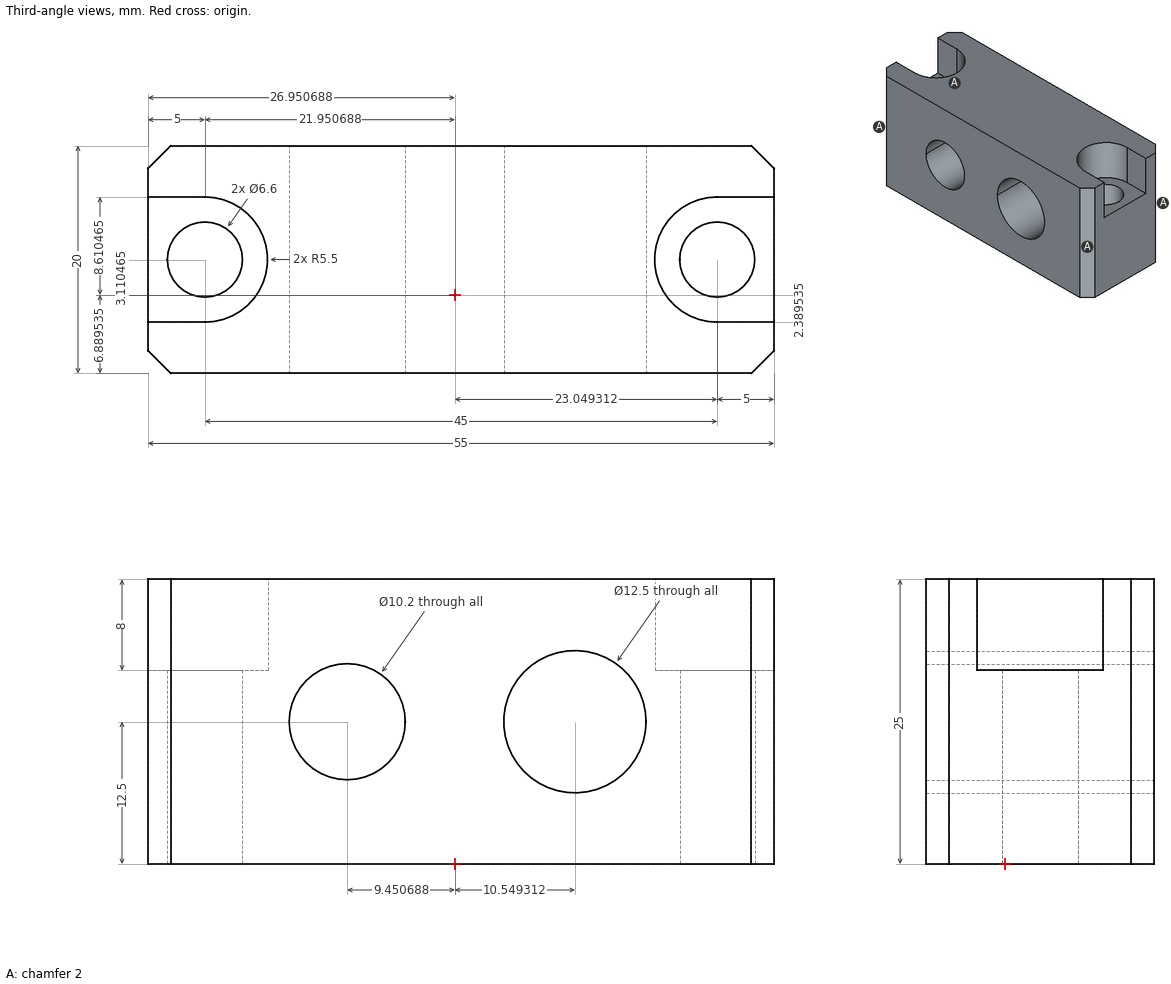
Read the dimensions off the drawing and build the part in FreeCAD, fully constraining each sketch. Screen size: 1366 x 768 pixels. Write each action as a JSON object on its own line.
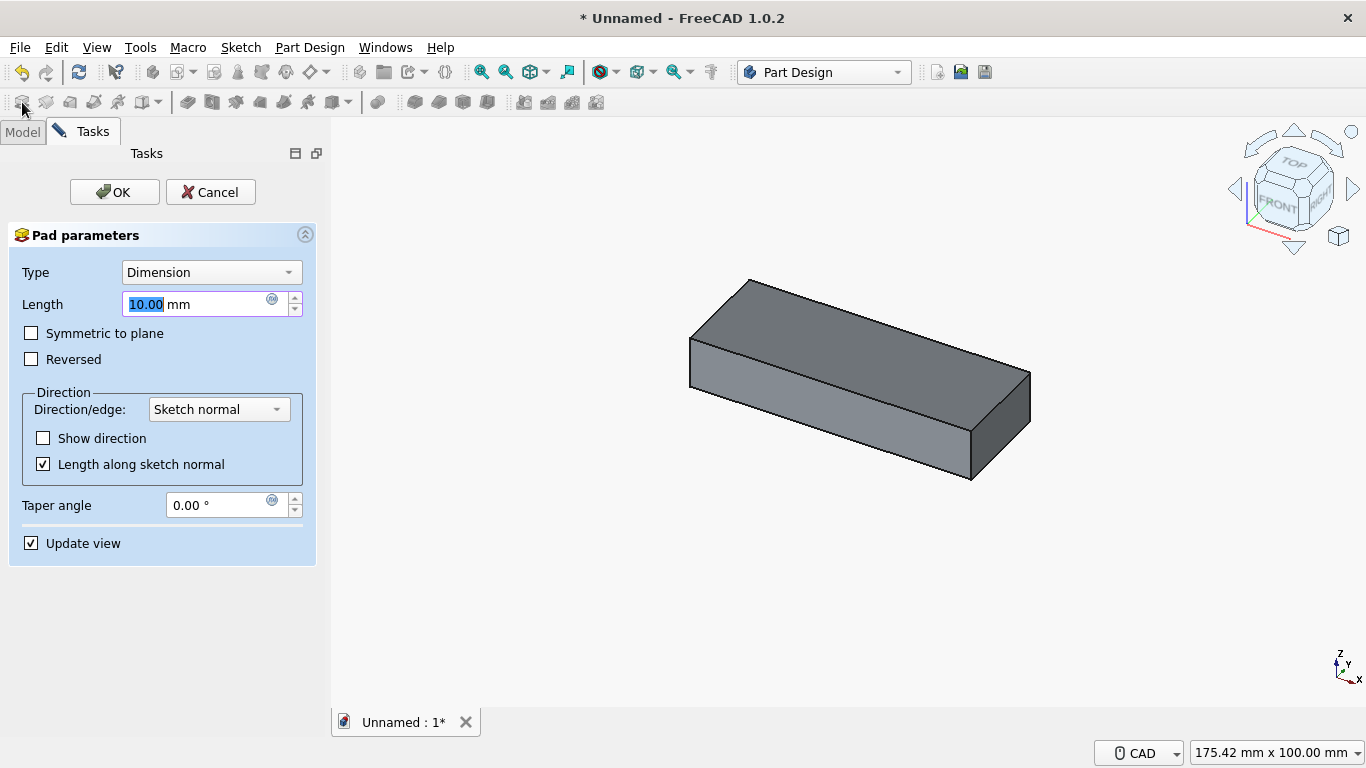
{"action": "type", "text": "25"}
{"action": "key", "text": "Tab"}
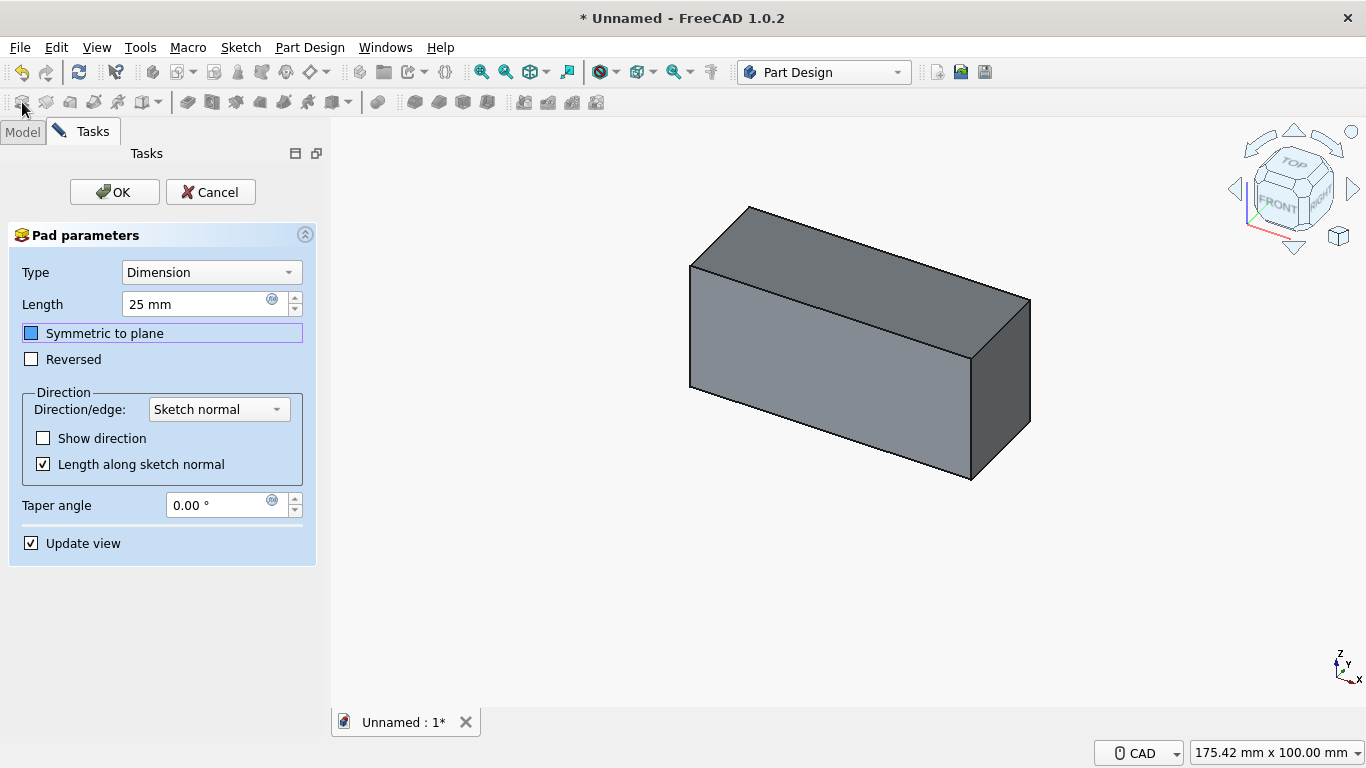
{"action": "left_click", "coordinate": [115, 192]}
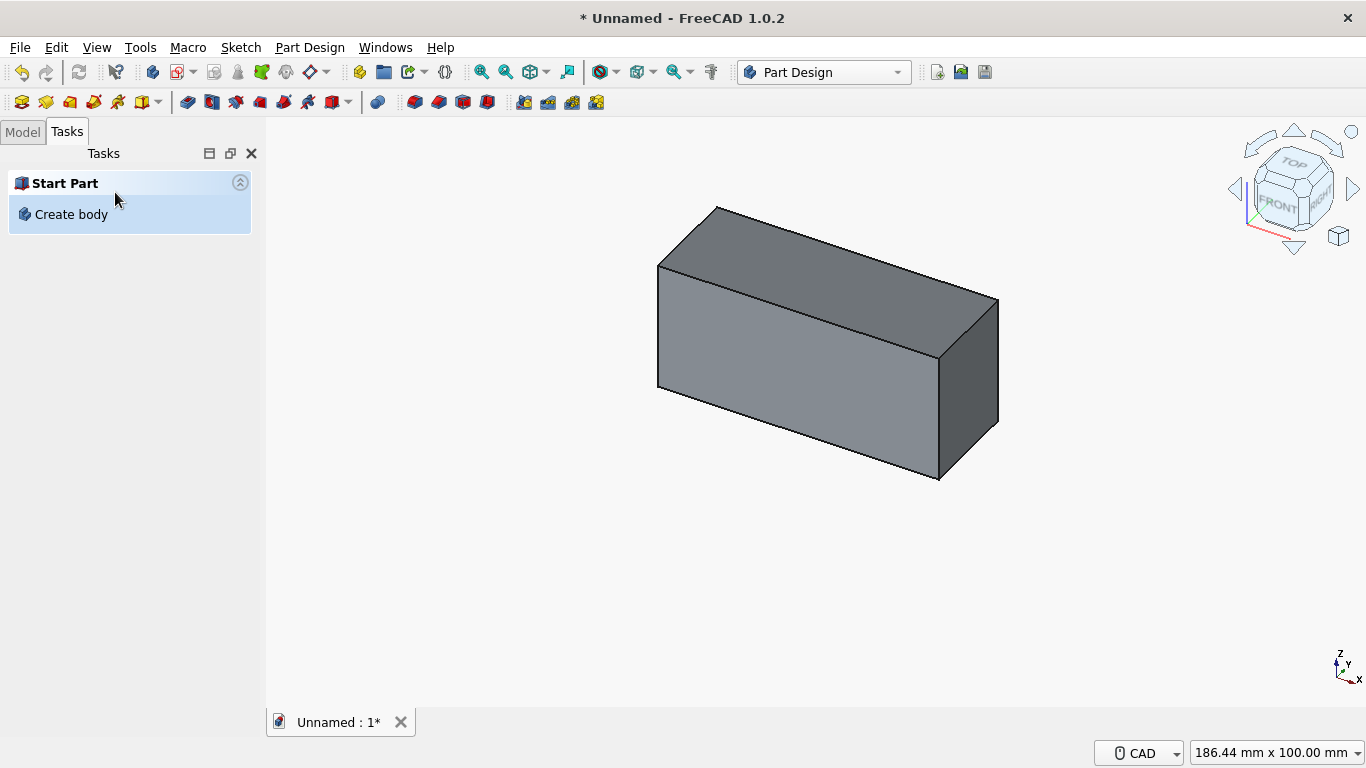
{"action": "left_click", "coordinate": [939, 418]}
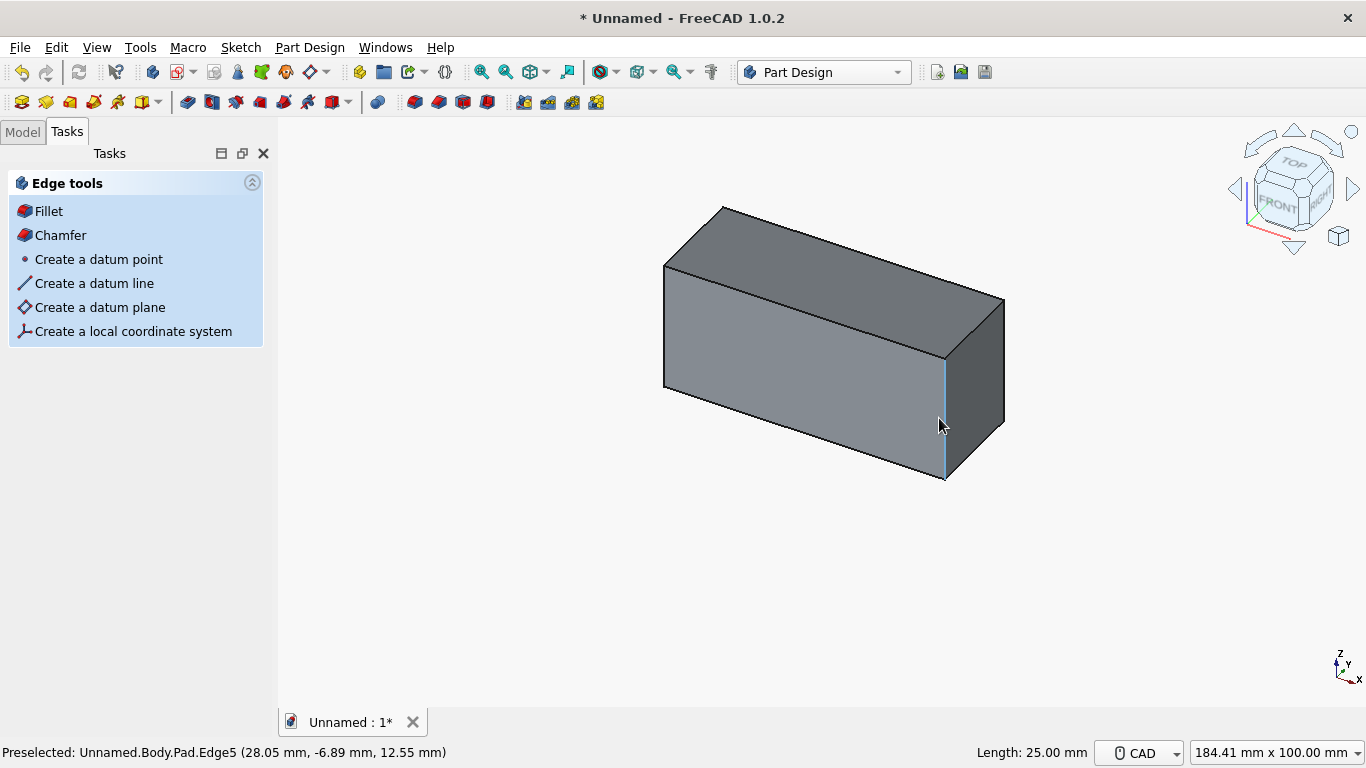
{"action": "key", "text": "0"}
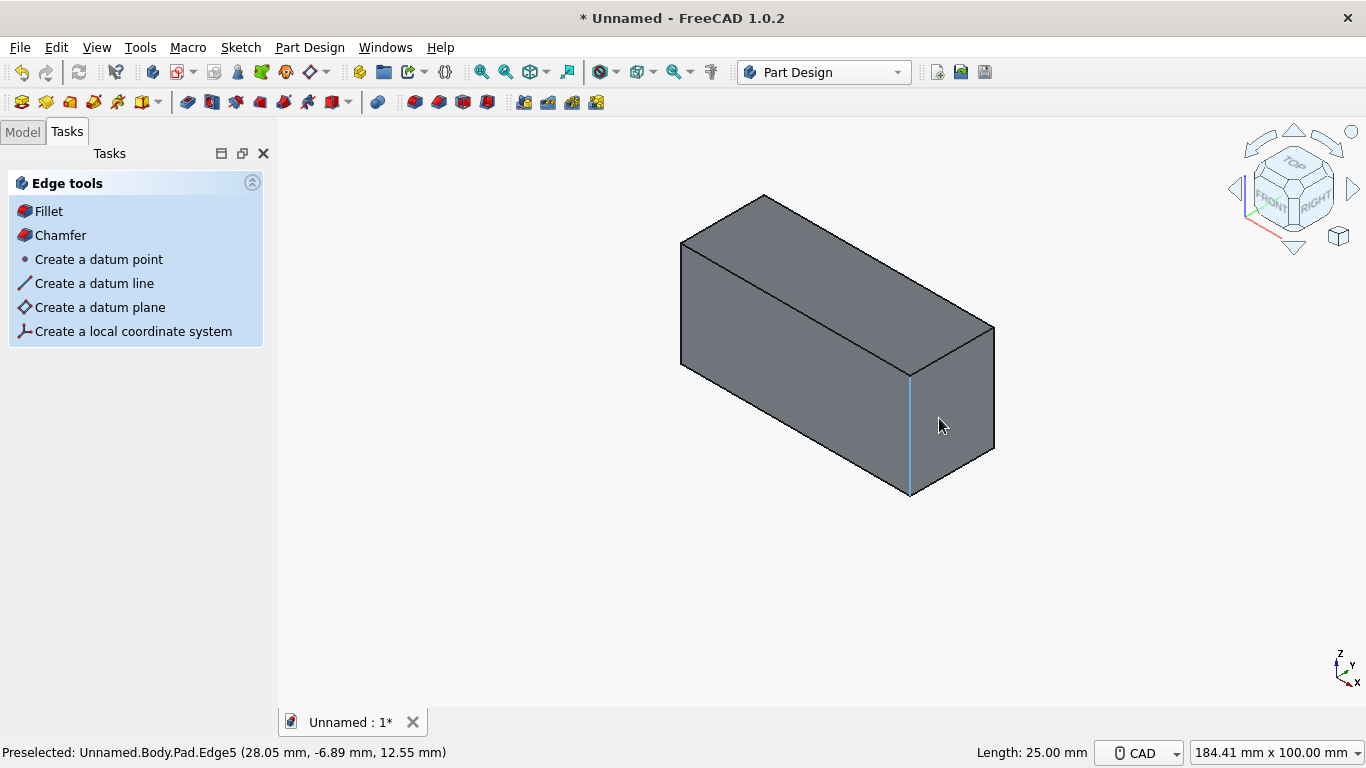
{"action": "key", "text": "2"}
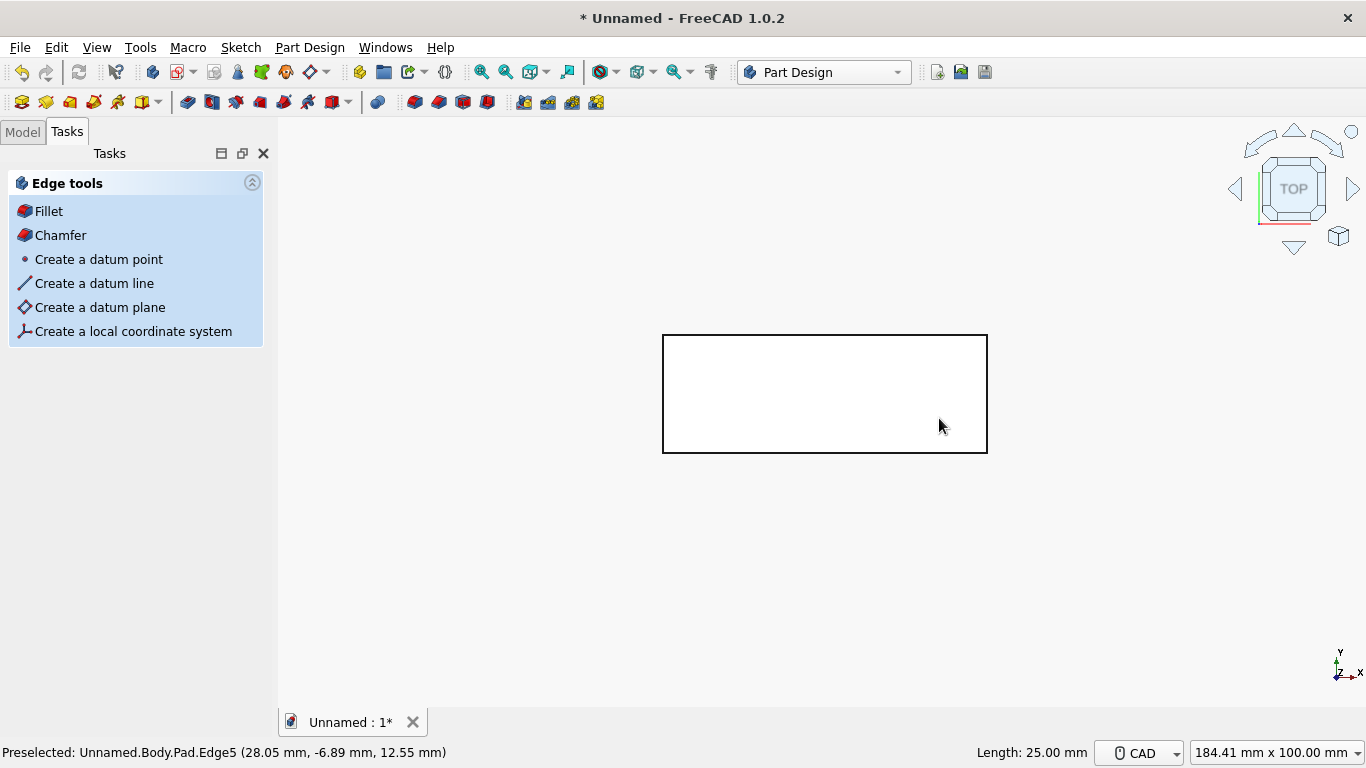
{"action": "left_click", "coordinate": [482, 72]}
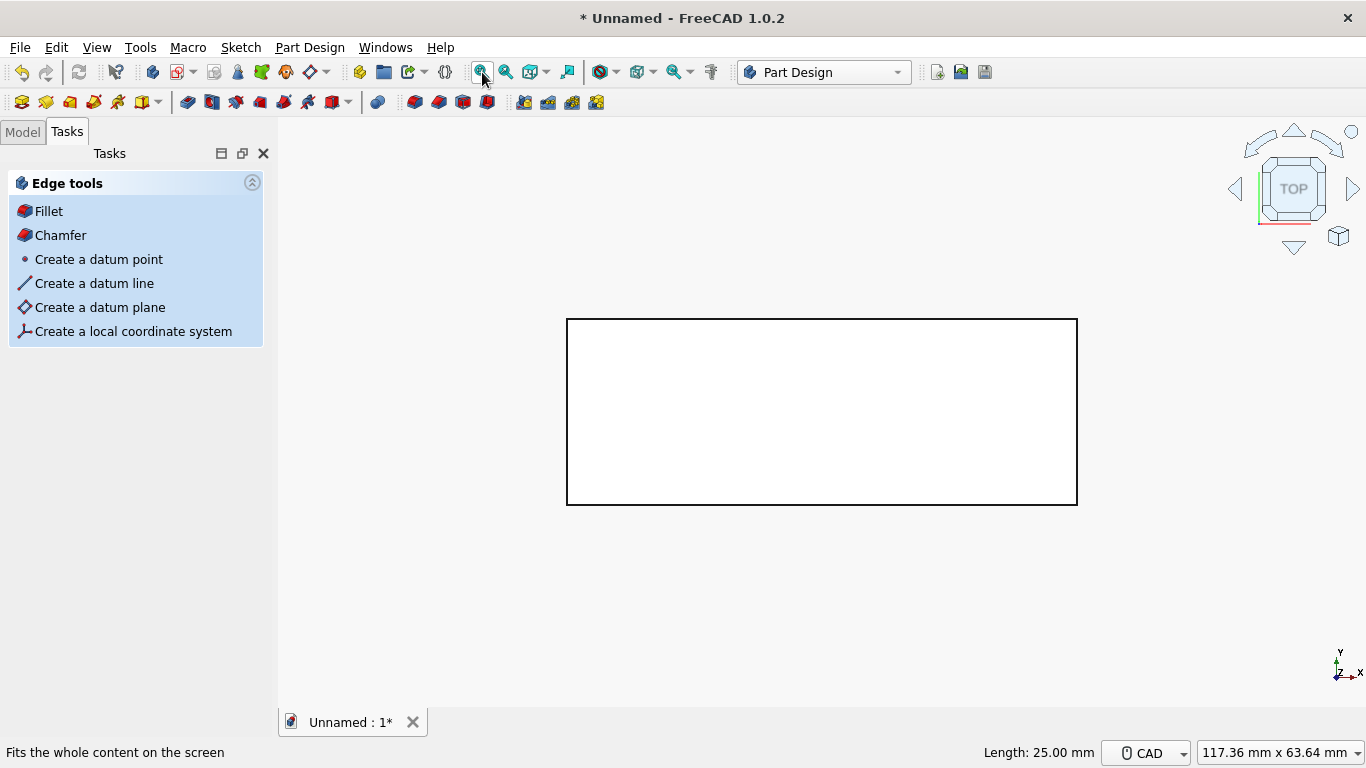
{"action": "key", "text": "1"}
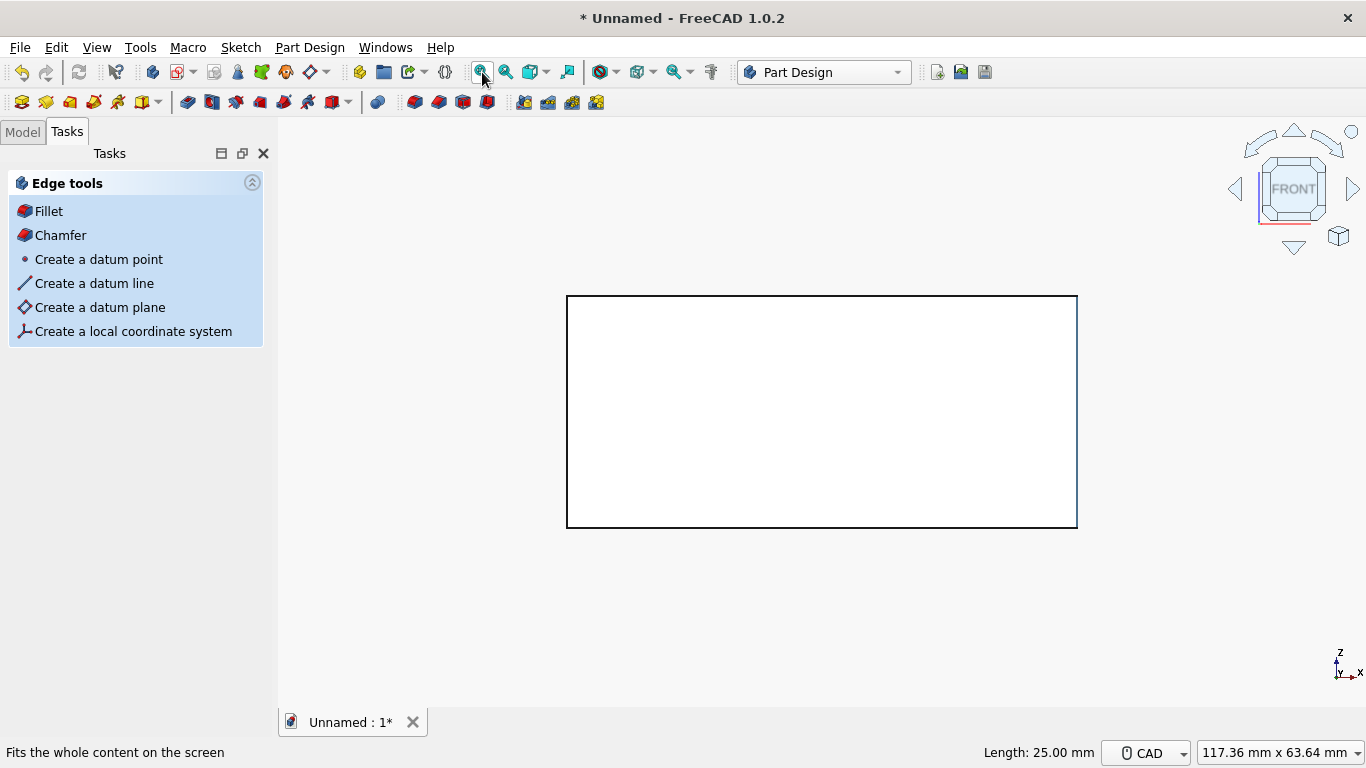
{"action": "left_click", "coordinate": [567, 411], "text": "ctrl"}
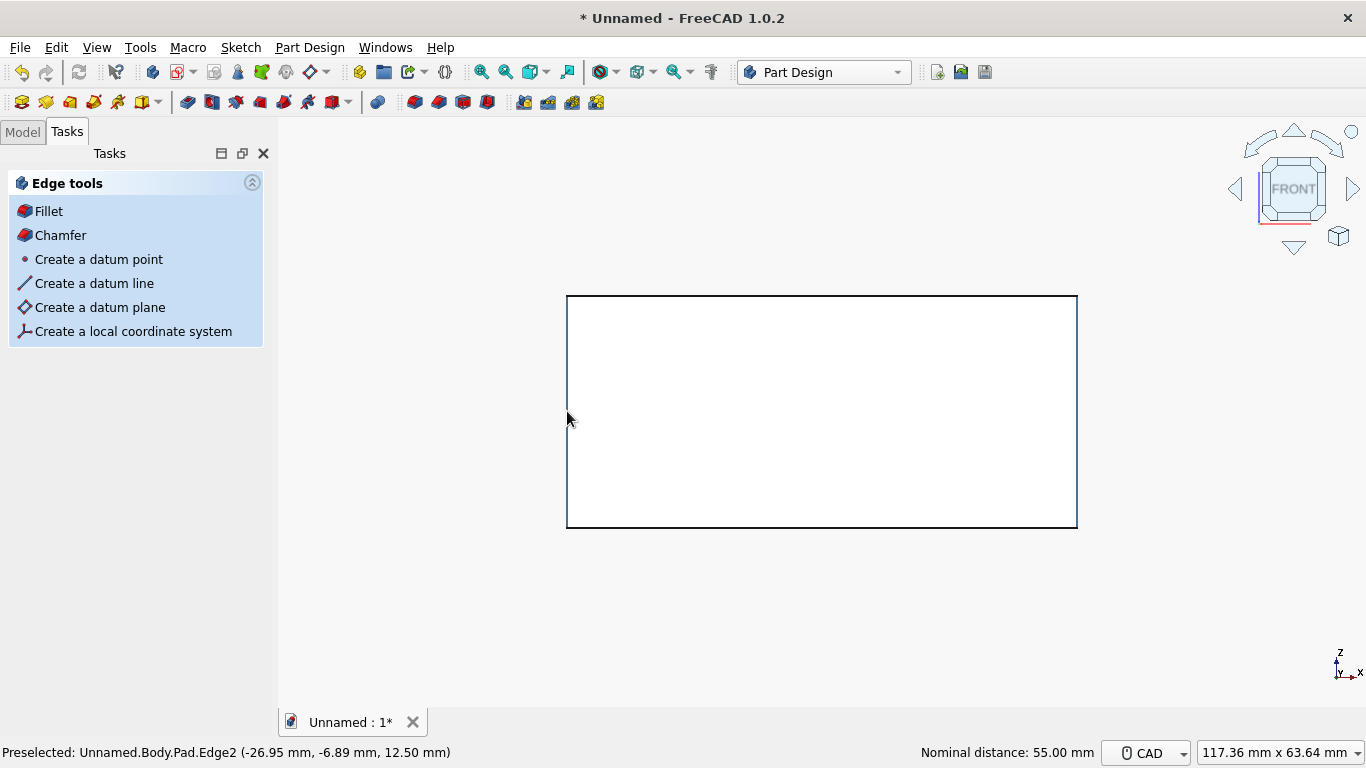
{"action": "key", "text": "3"}